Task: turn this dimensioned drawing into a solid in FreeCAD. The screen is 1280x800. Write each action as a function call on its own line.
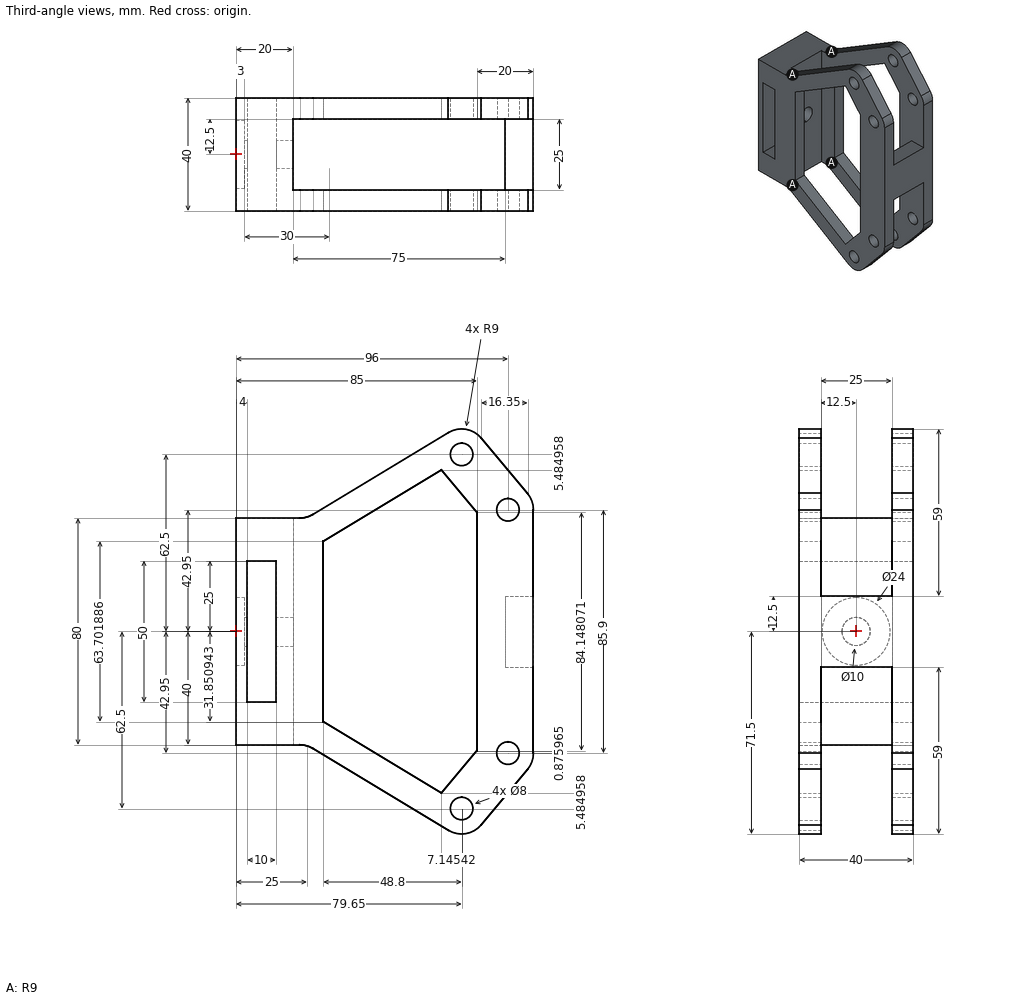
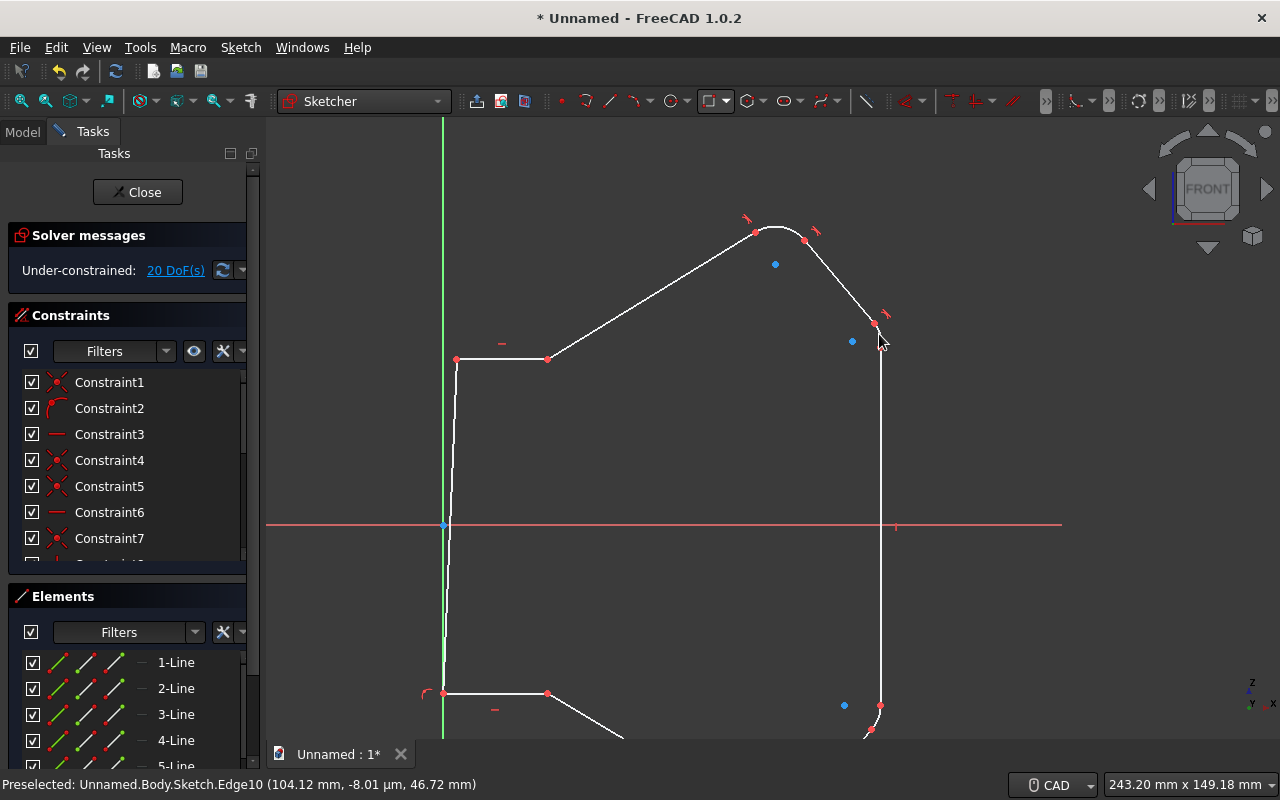
click(881, 455)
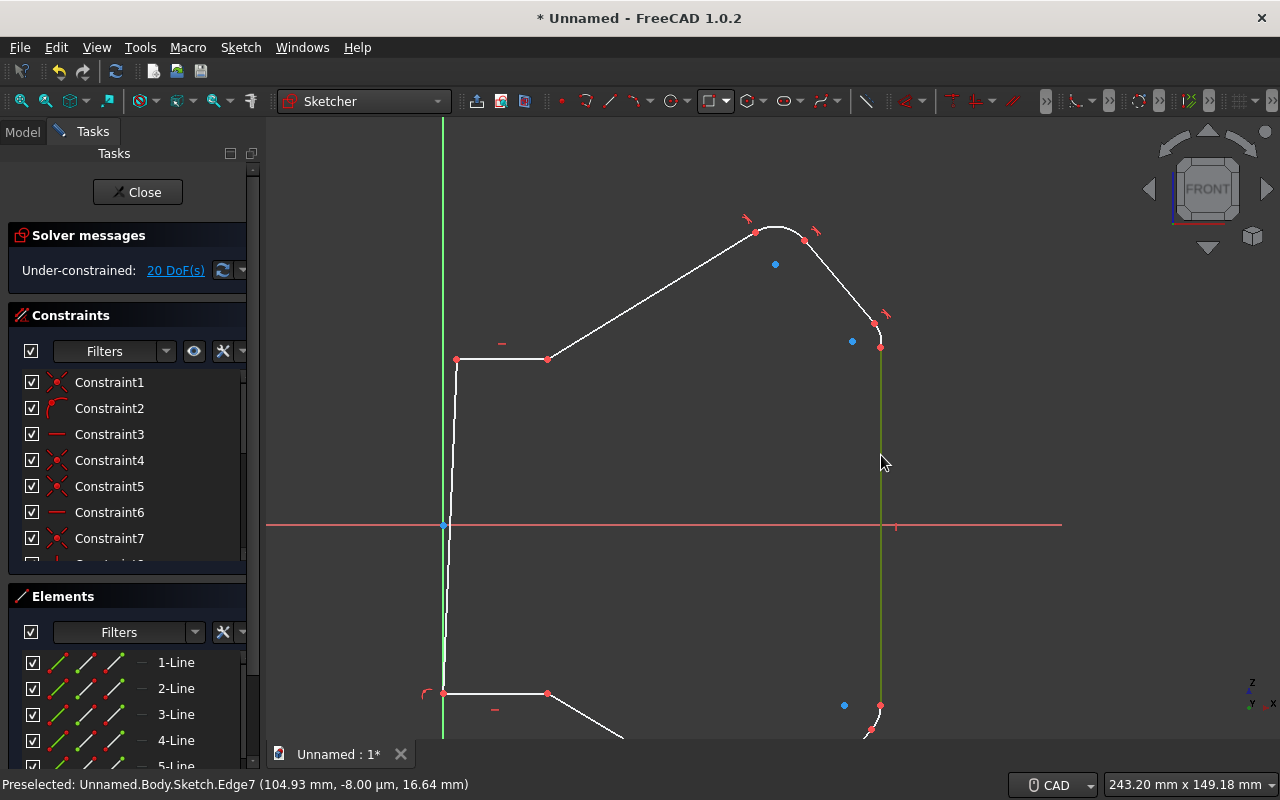
click(880, 335)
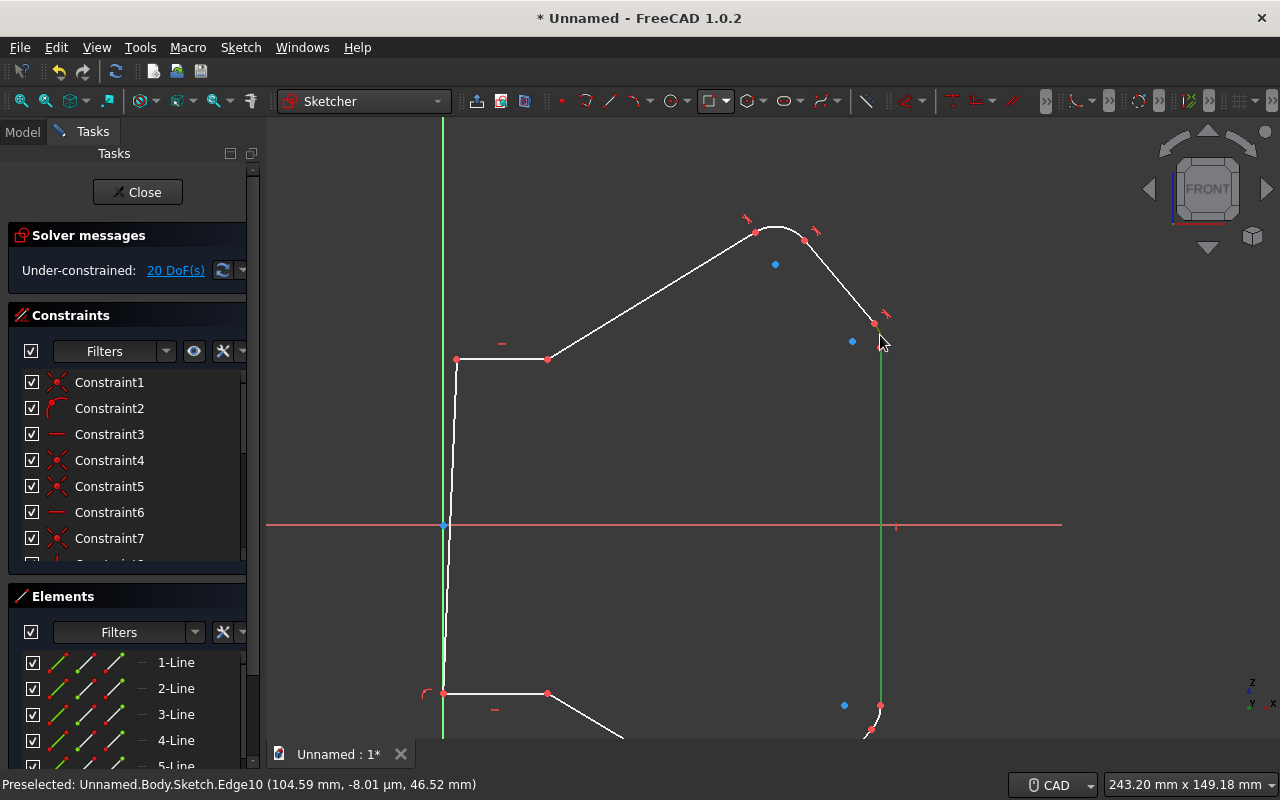
key(t)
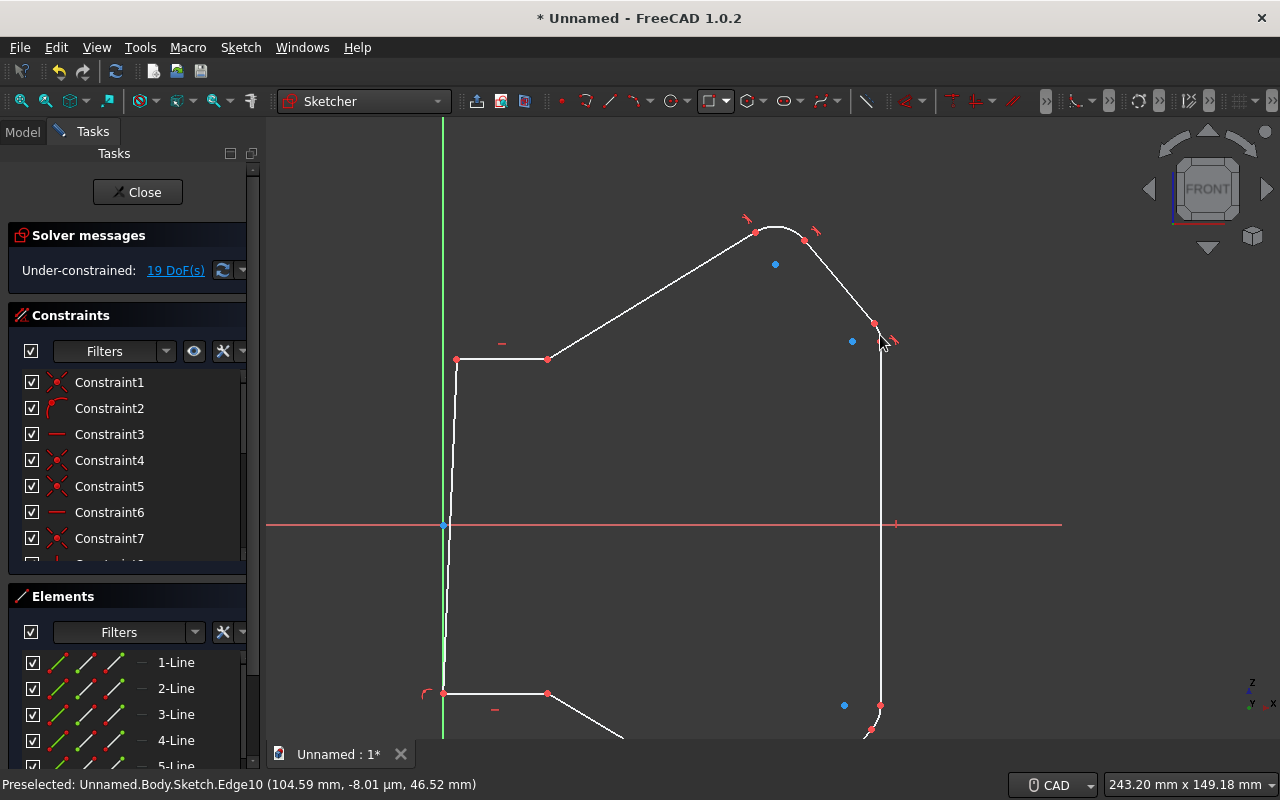
click(881, 451)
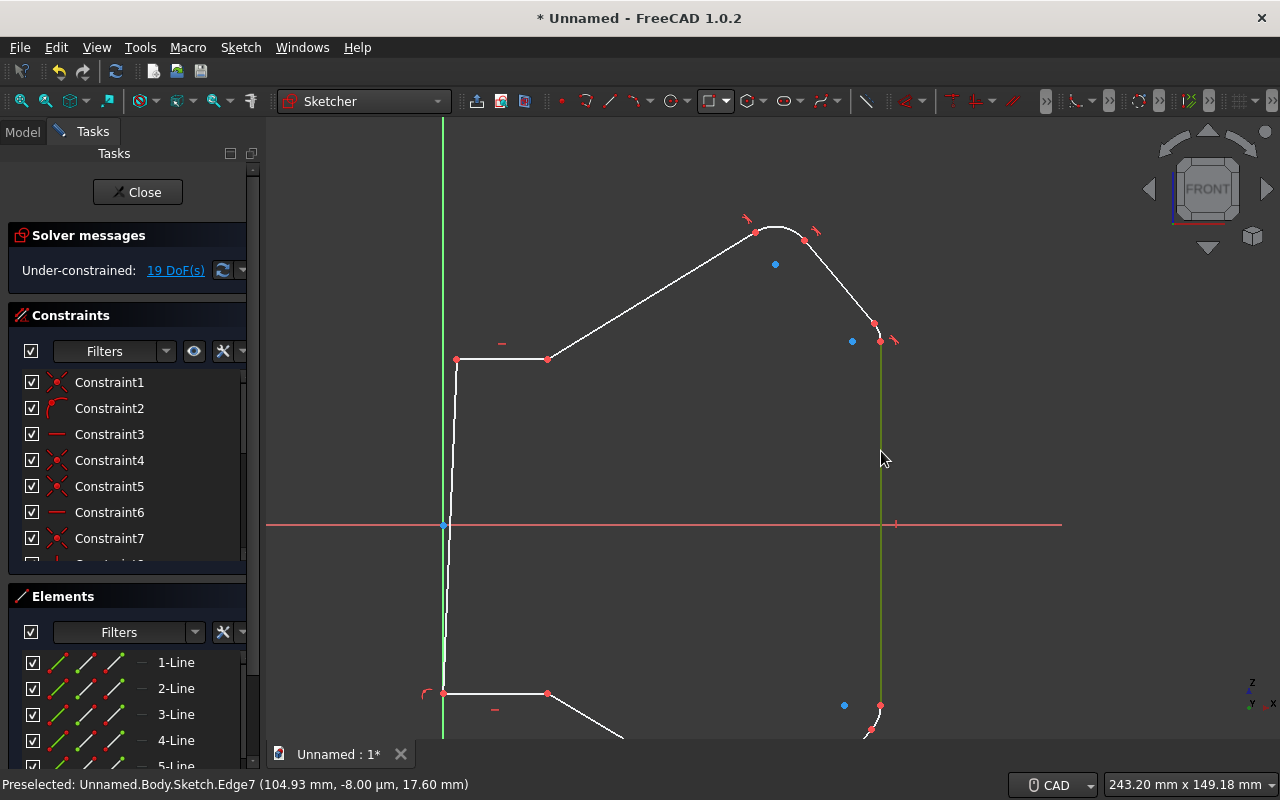
scroll(791, 230, down, 2)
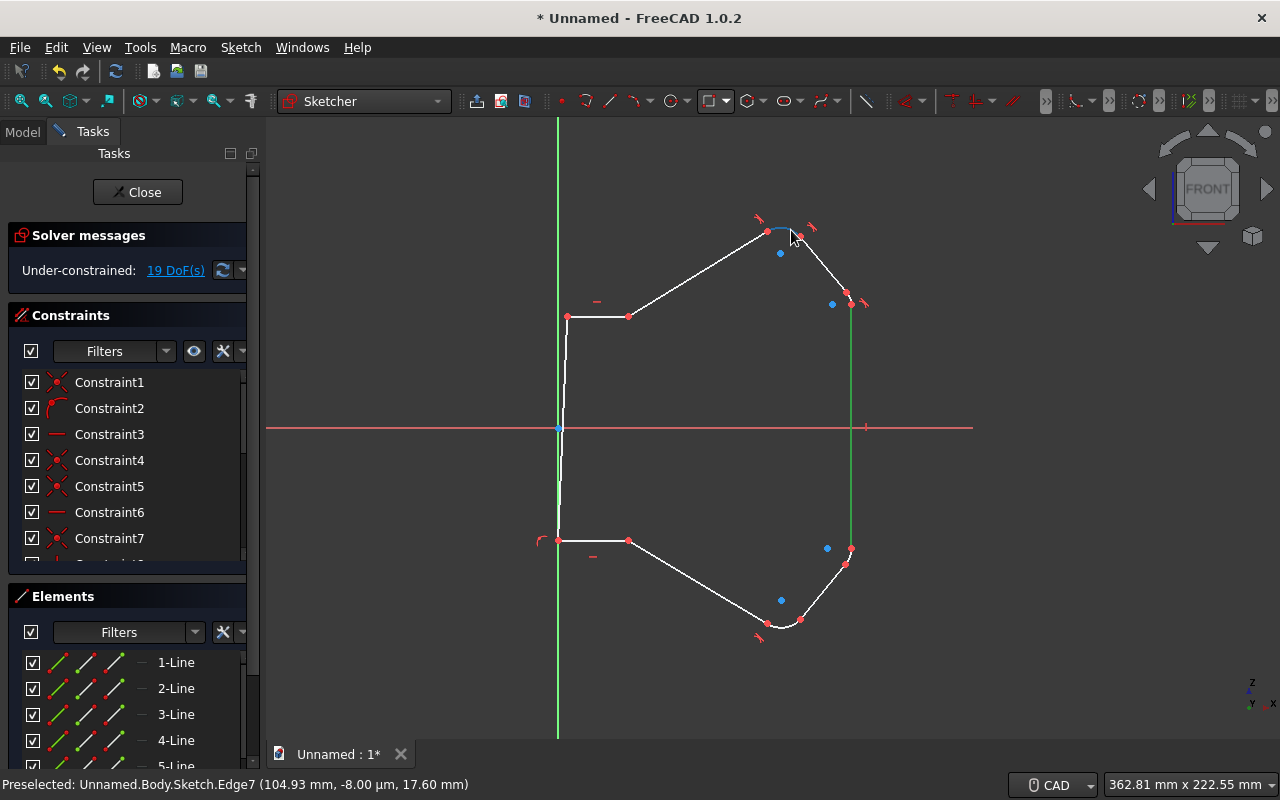
scroll(850, 557, up, 3)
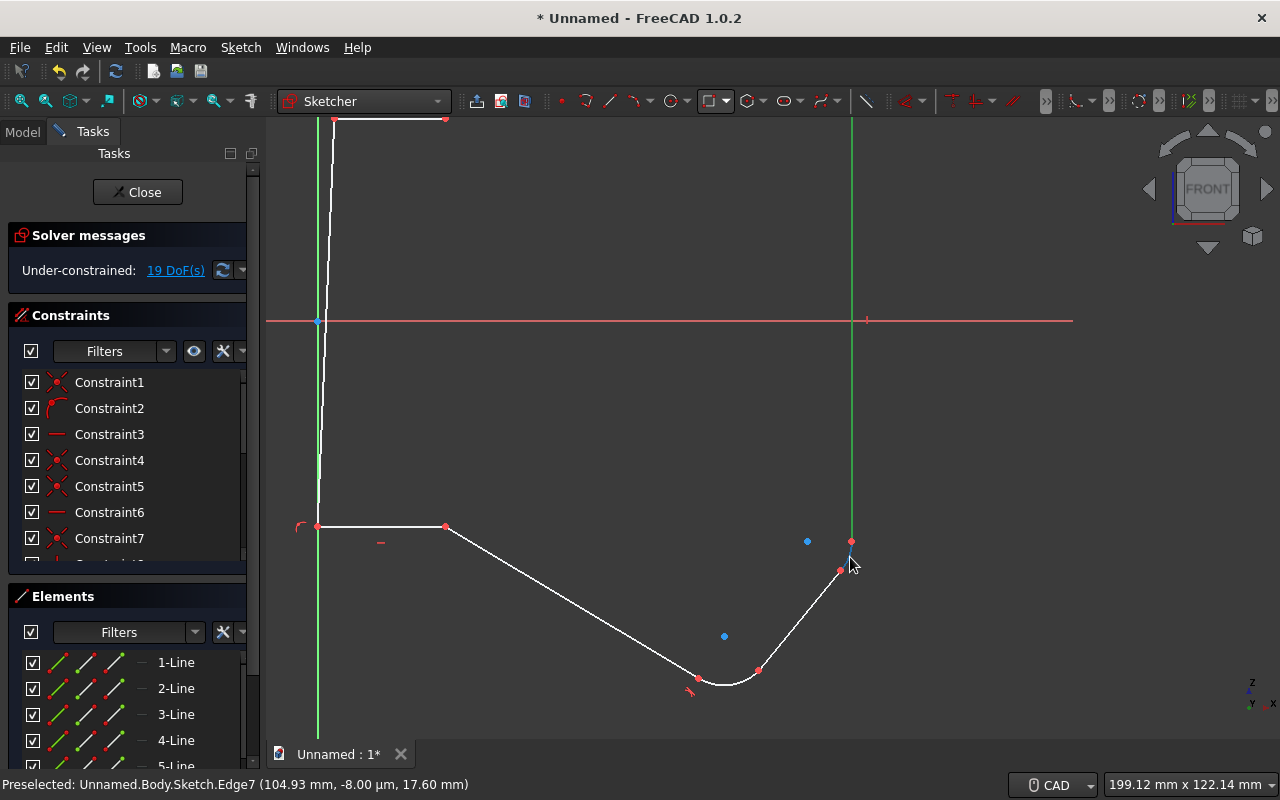
click(849, 557)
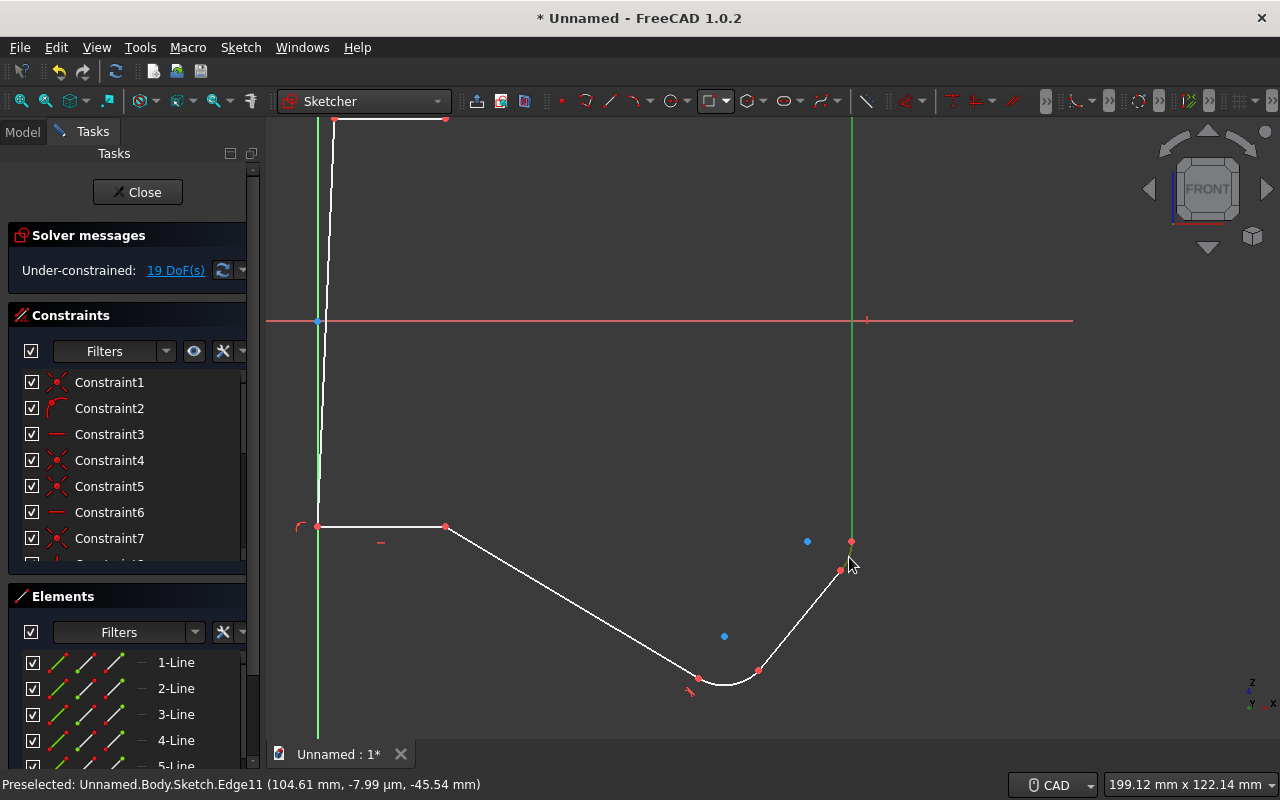
key(t)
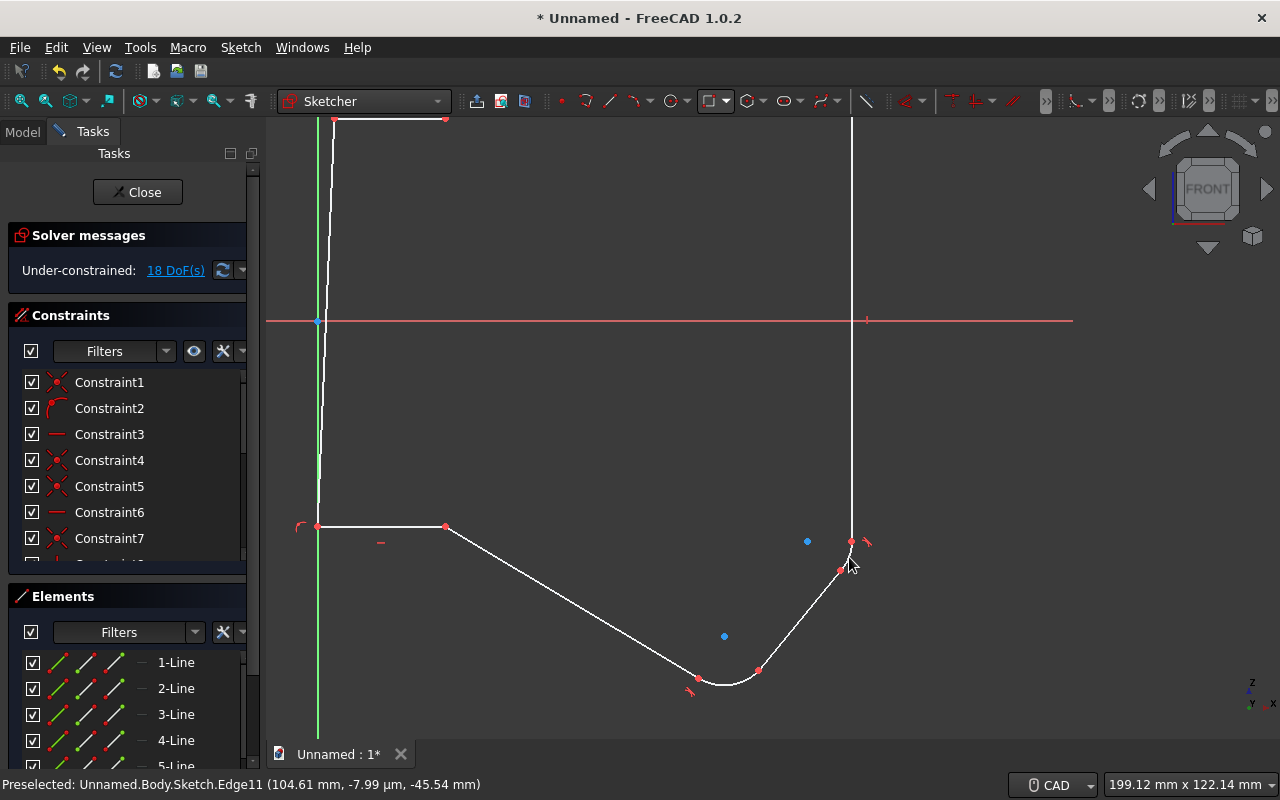
click(816, 601)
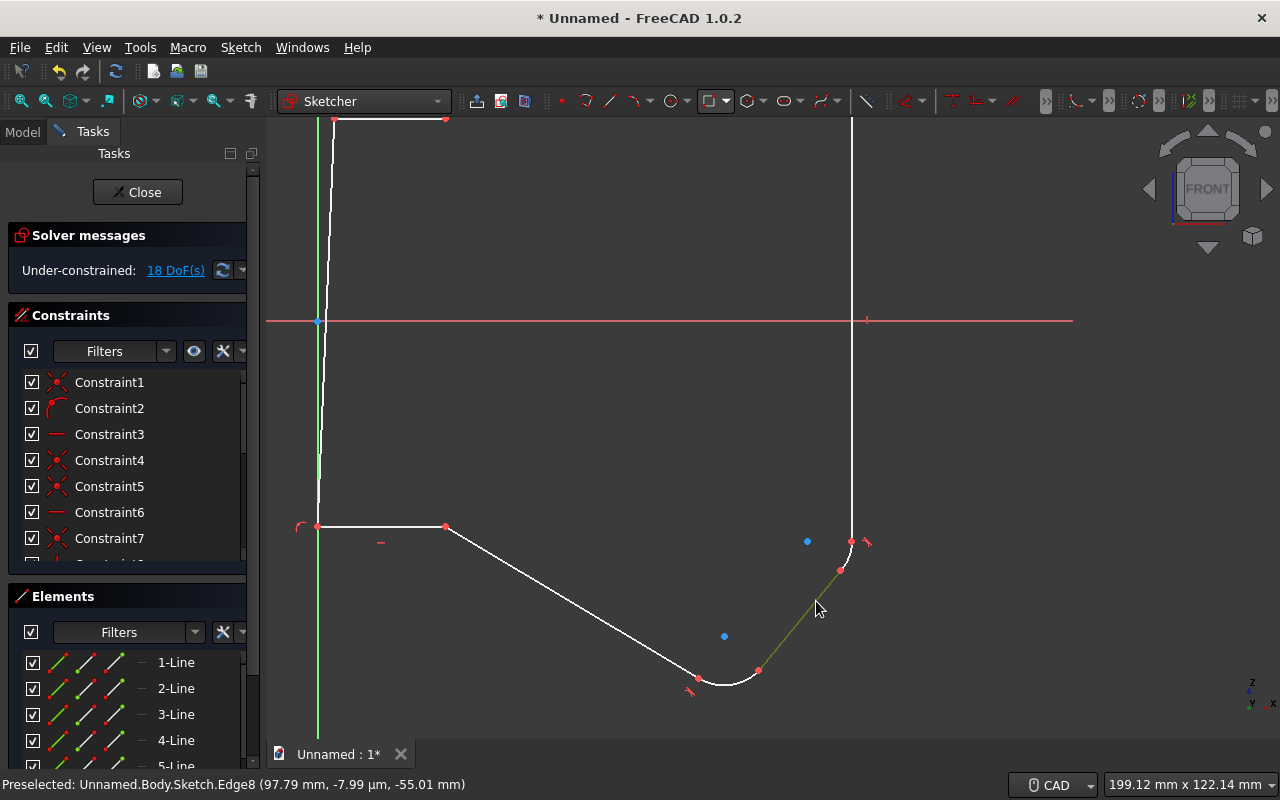
scroll(846, 563, up, 2)